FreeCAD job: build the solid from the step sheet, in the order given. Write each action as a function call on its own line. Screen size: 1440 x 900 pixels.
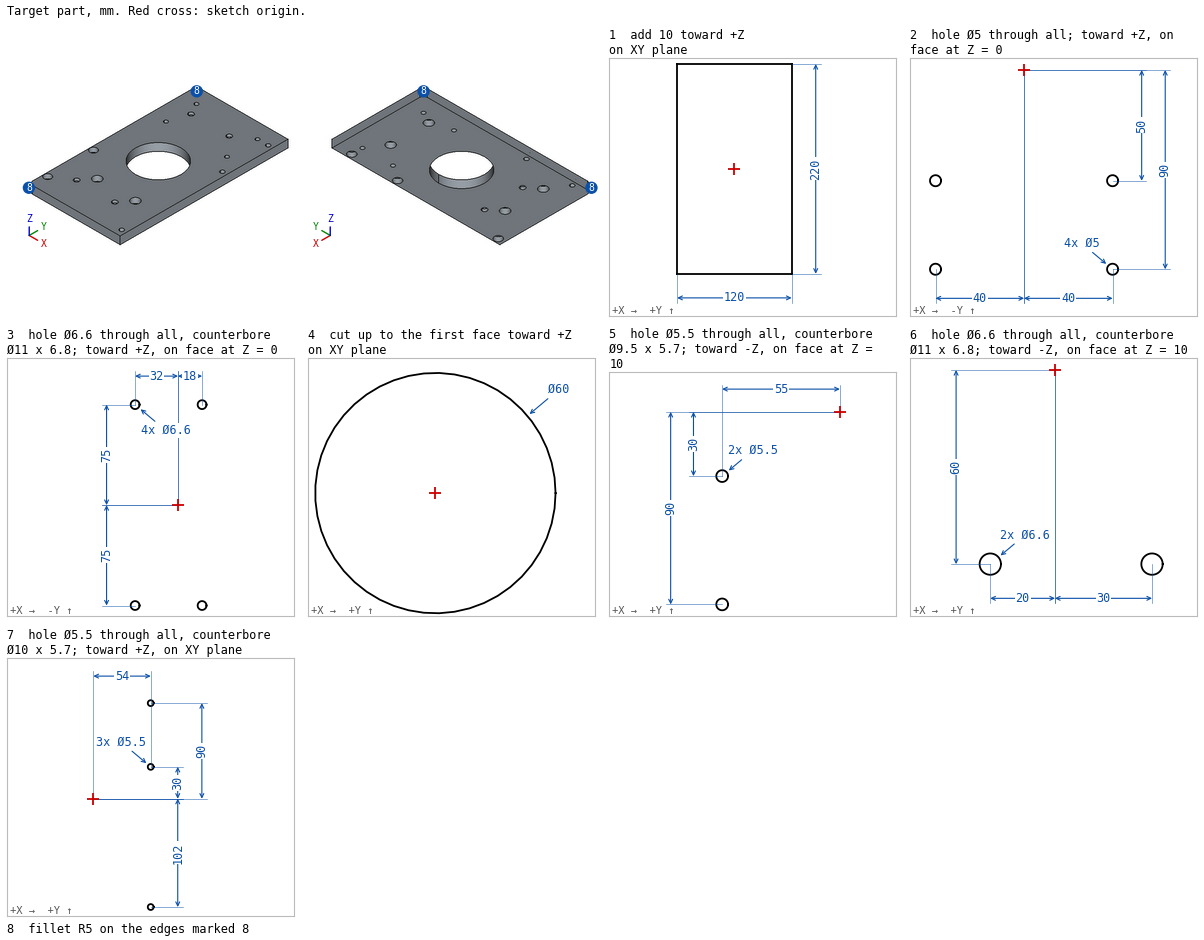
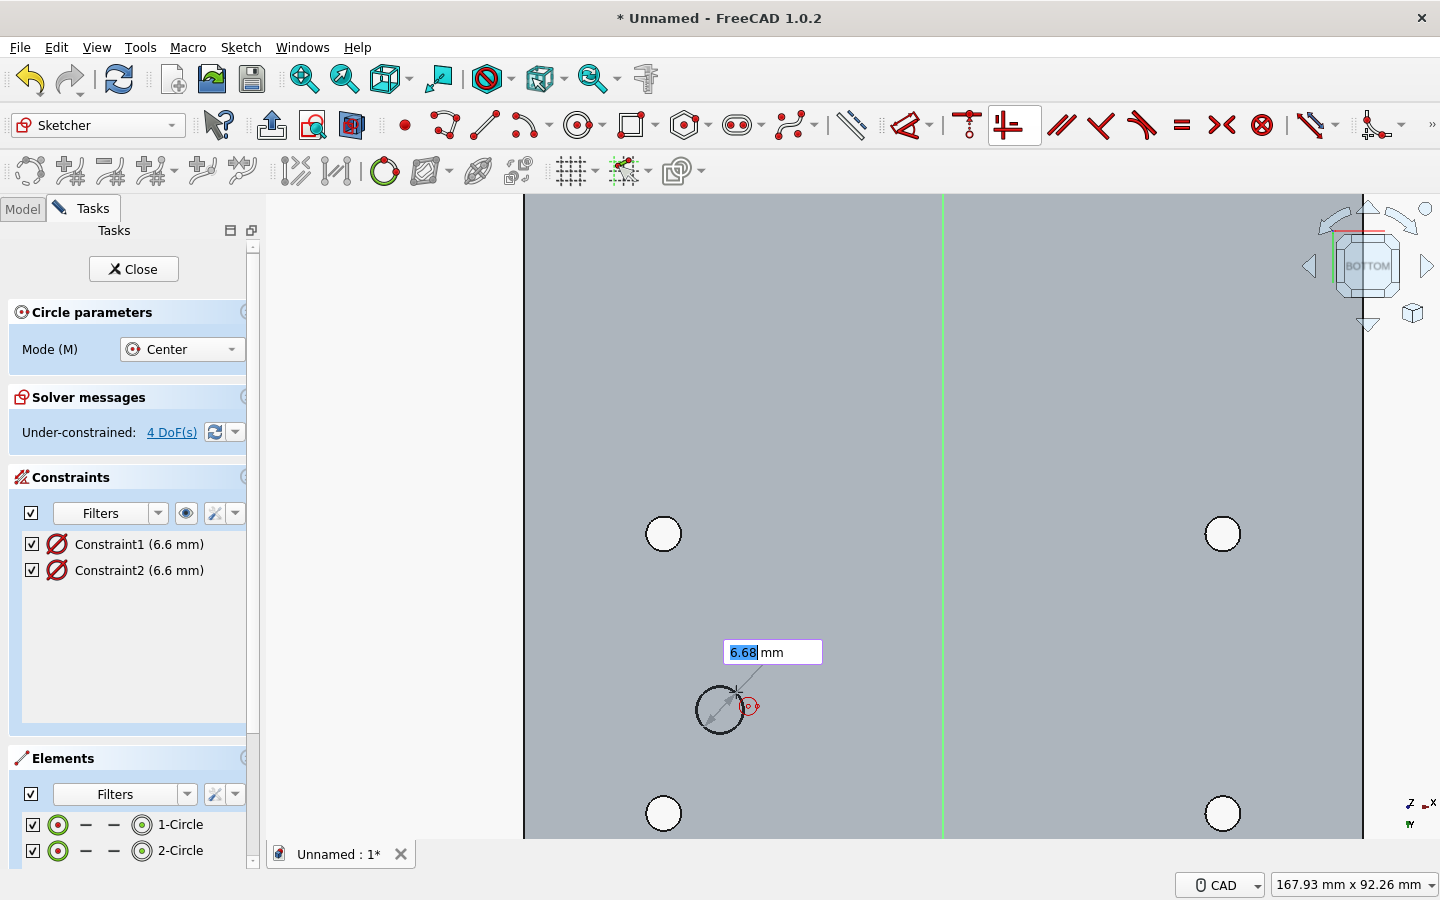
text(6.6)
key(Return)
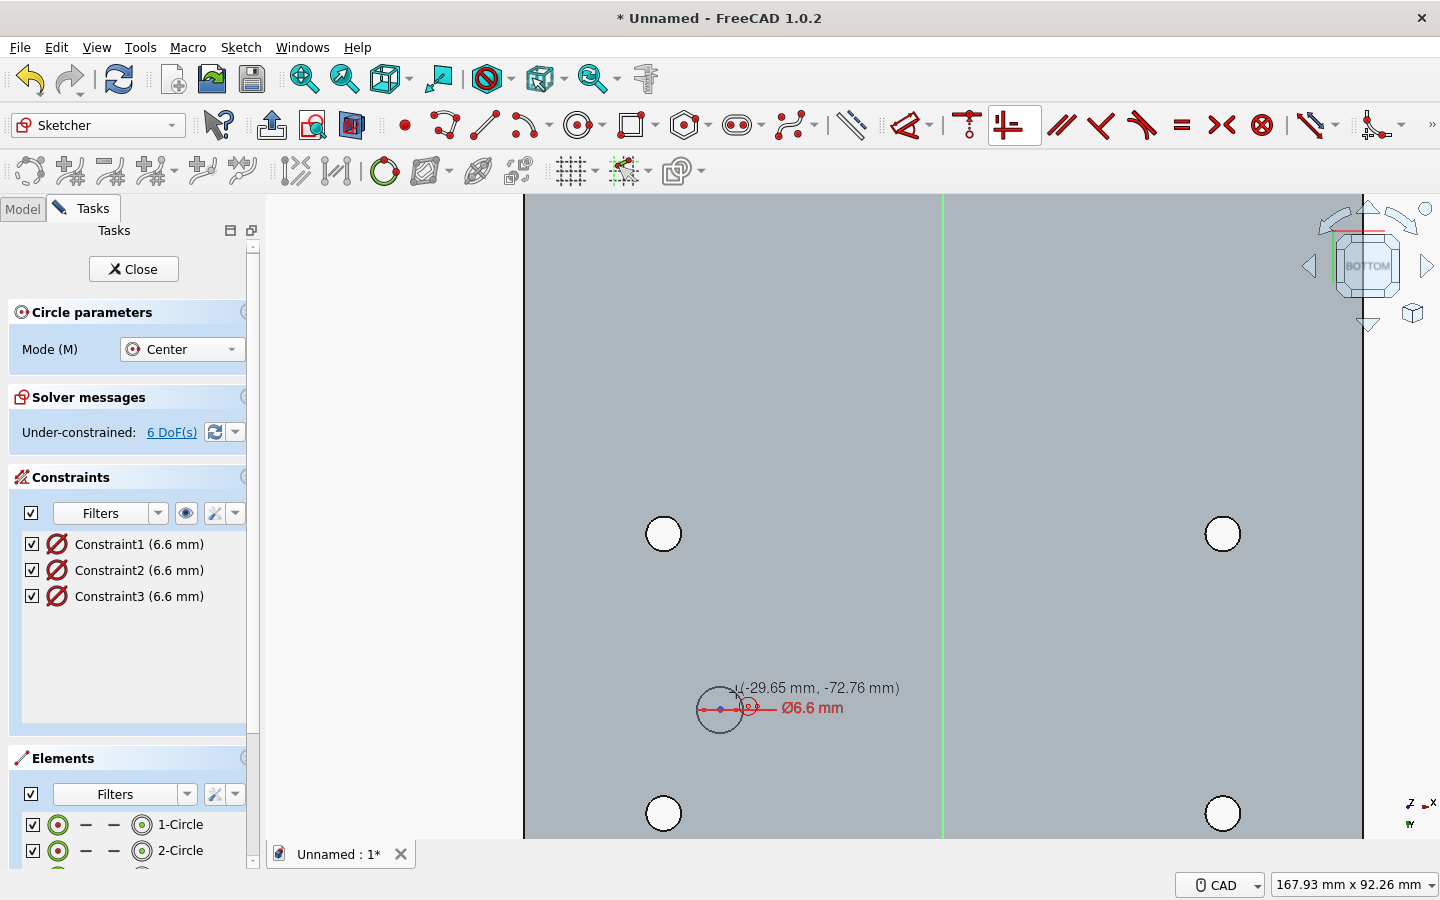
click(1069, 709)
move(1085, 692)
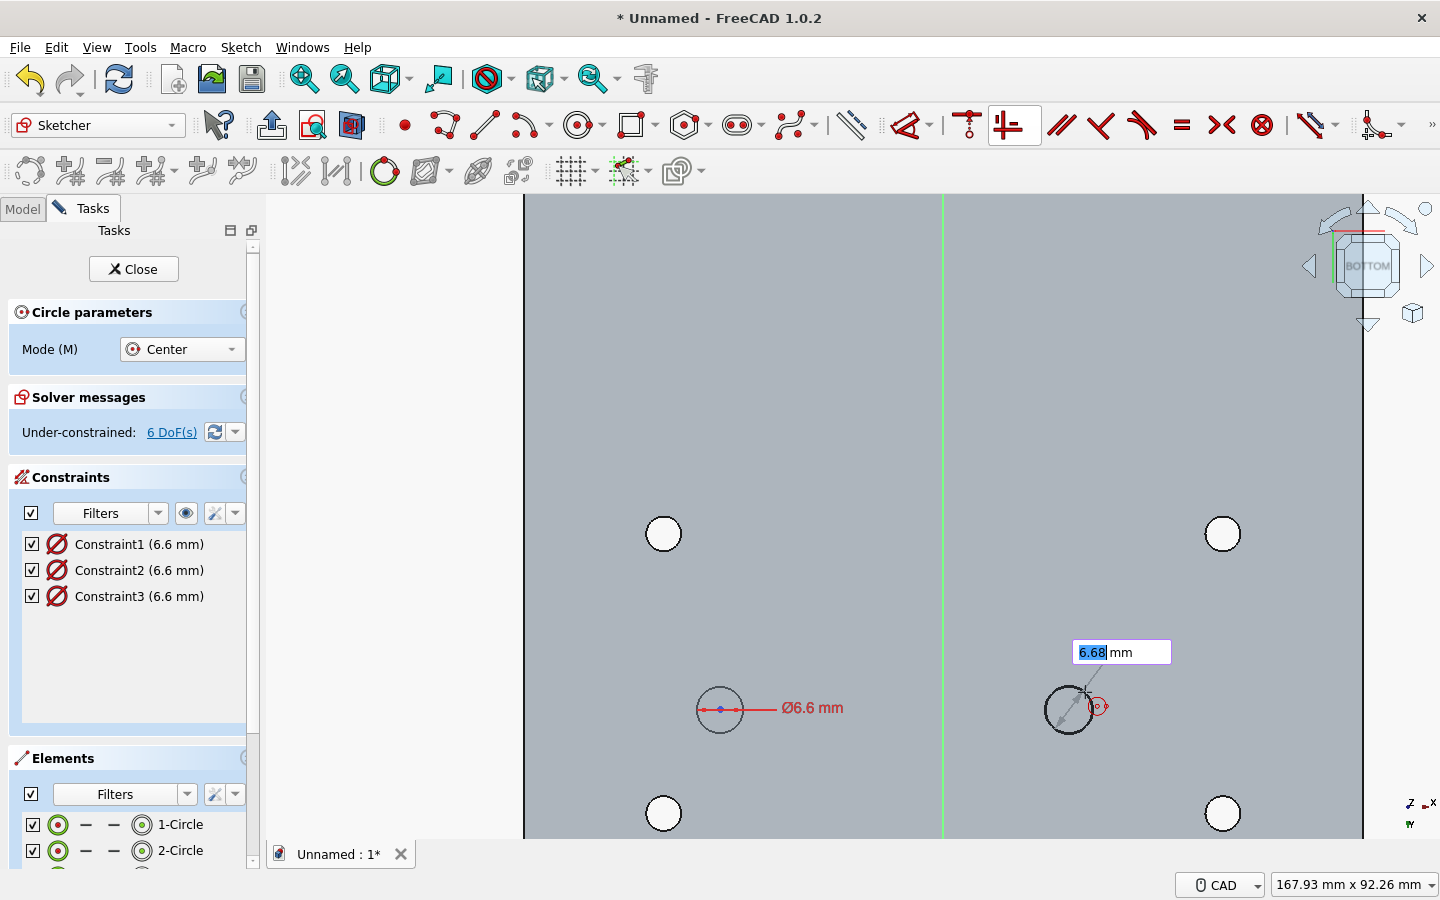
text(6.6)
key(Return)
key(Escape)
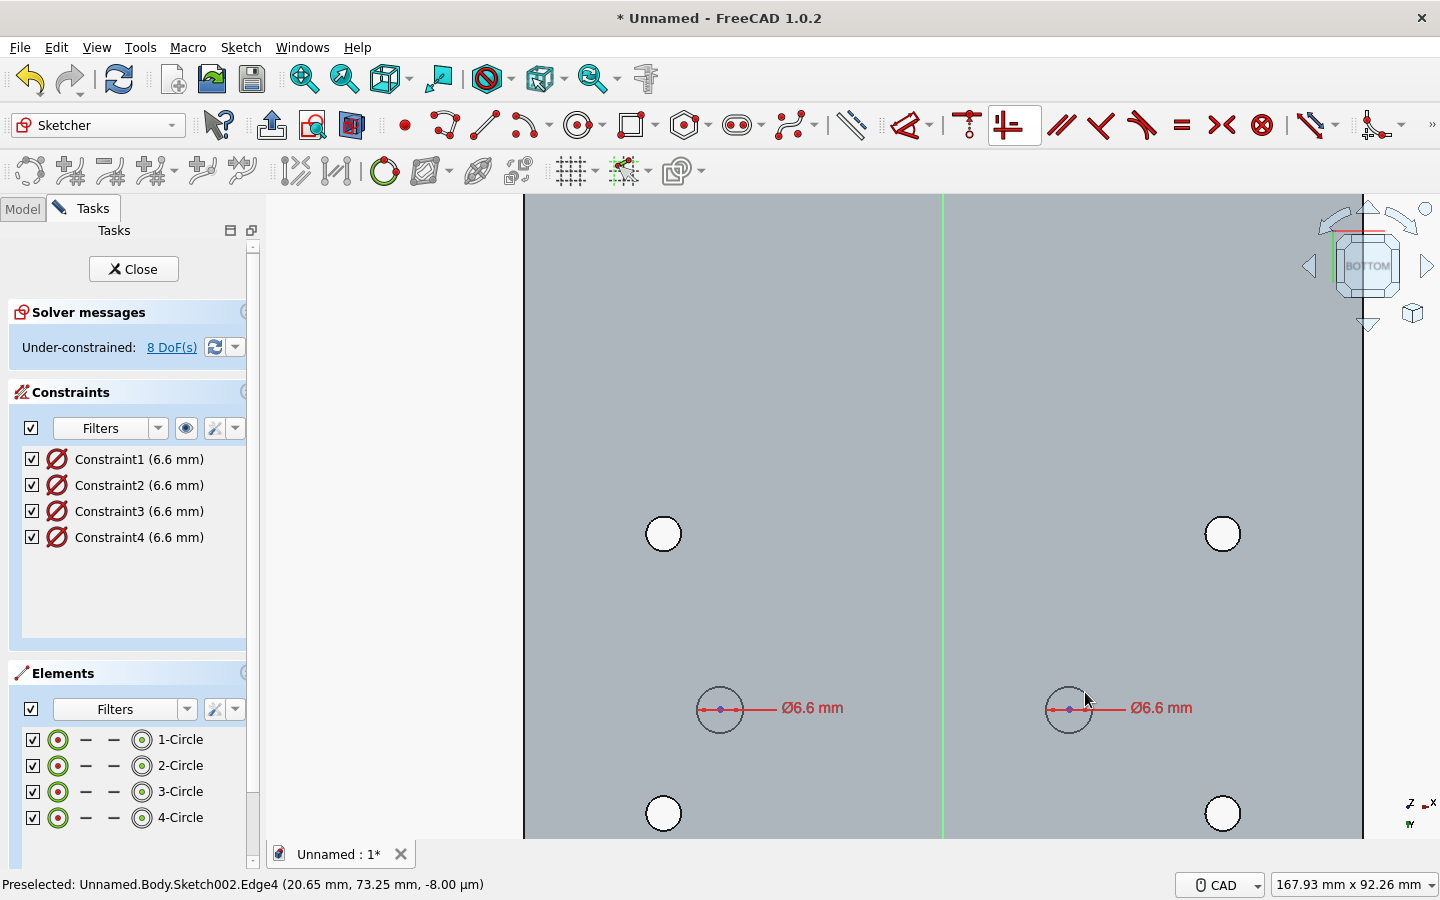
scroll(721, 710, down, 5)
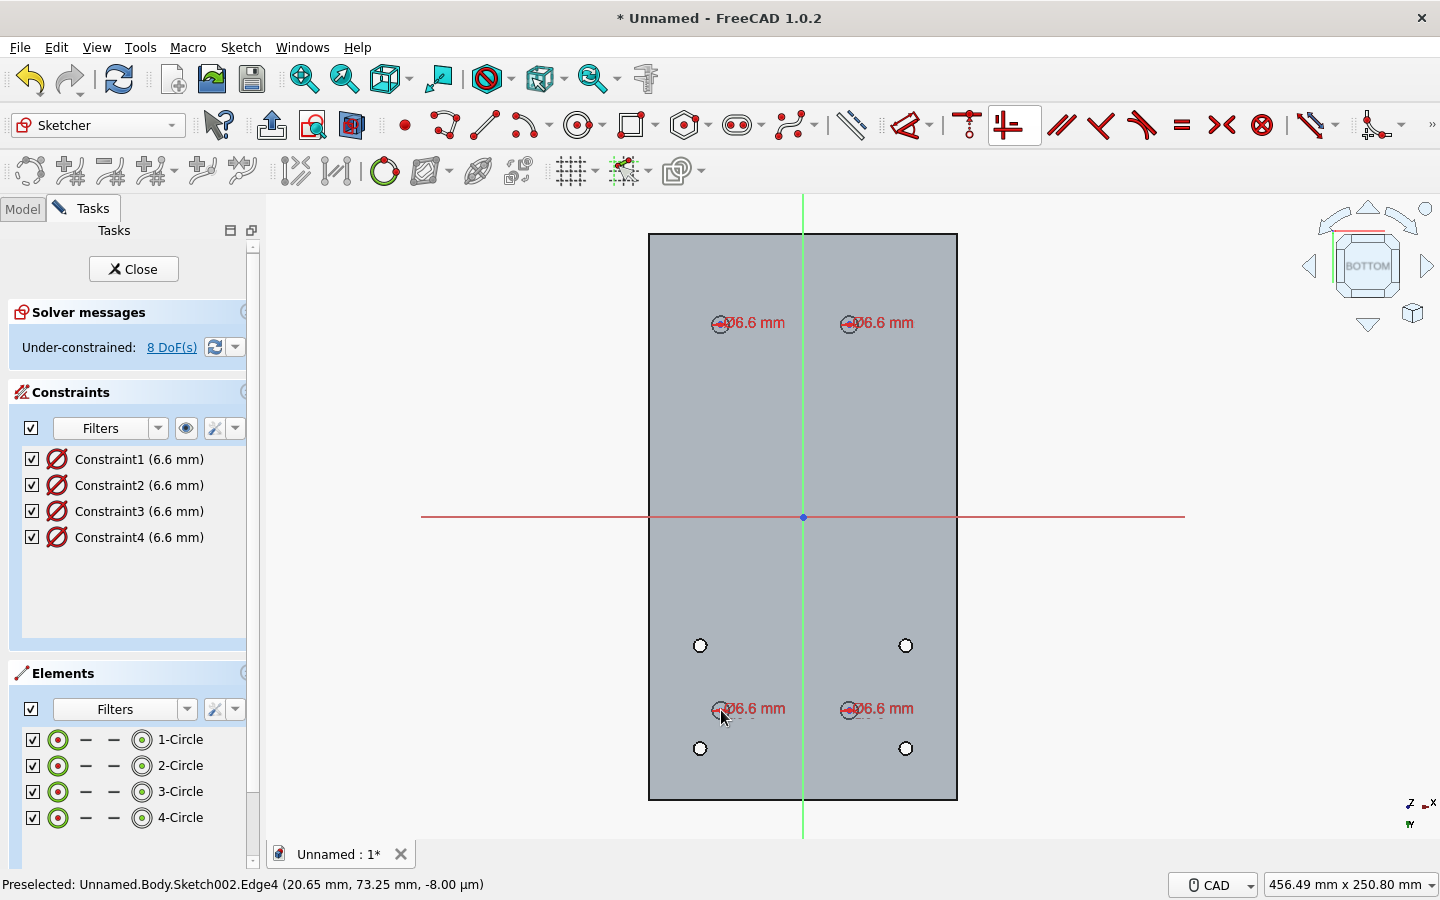
click(721, 325)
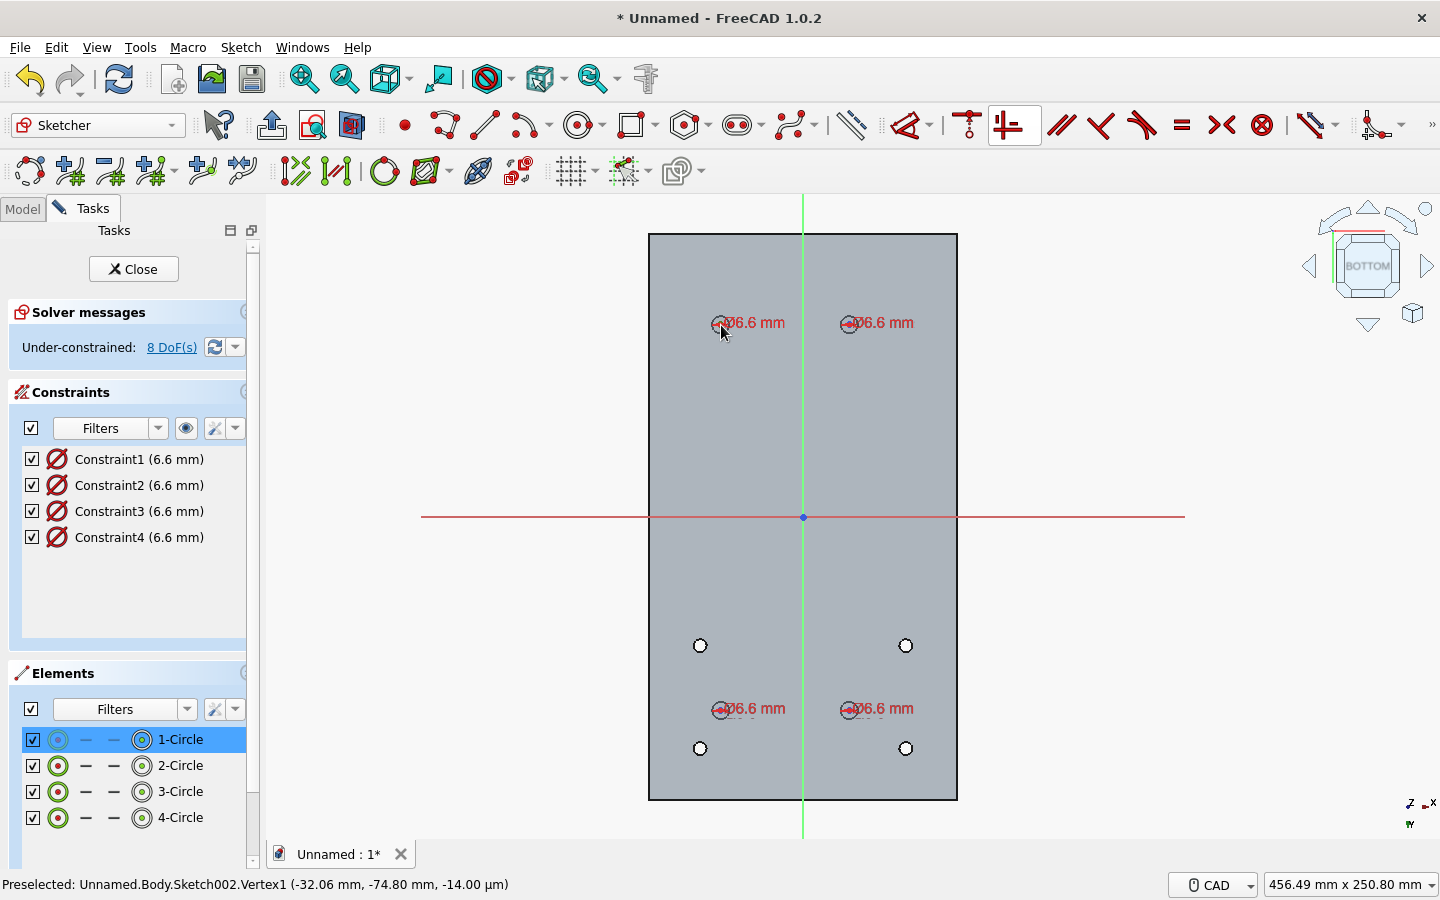
click(849, 325)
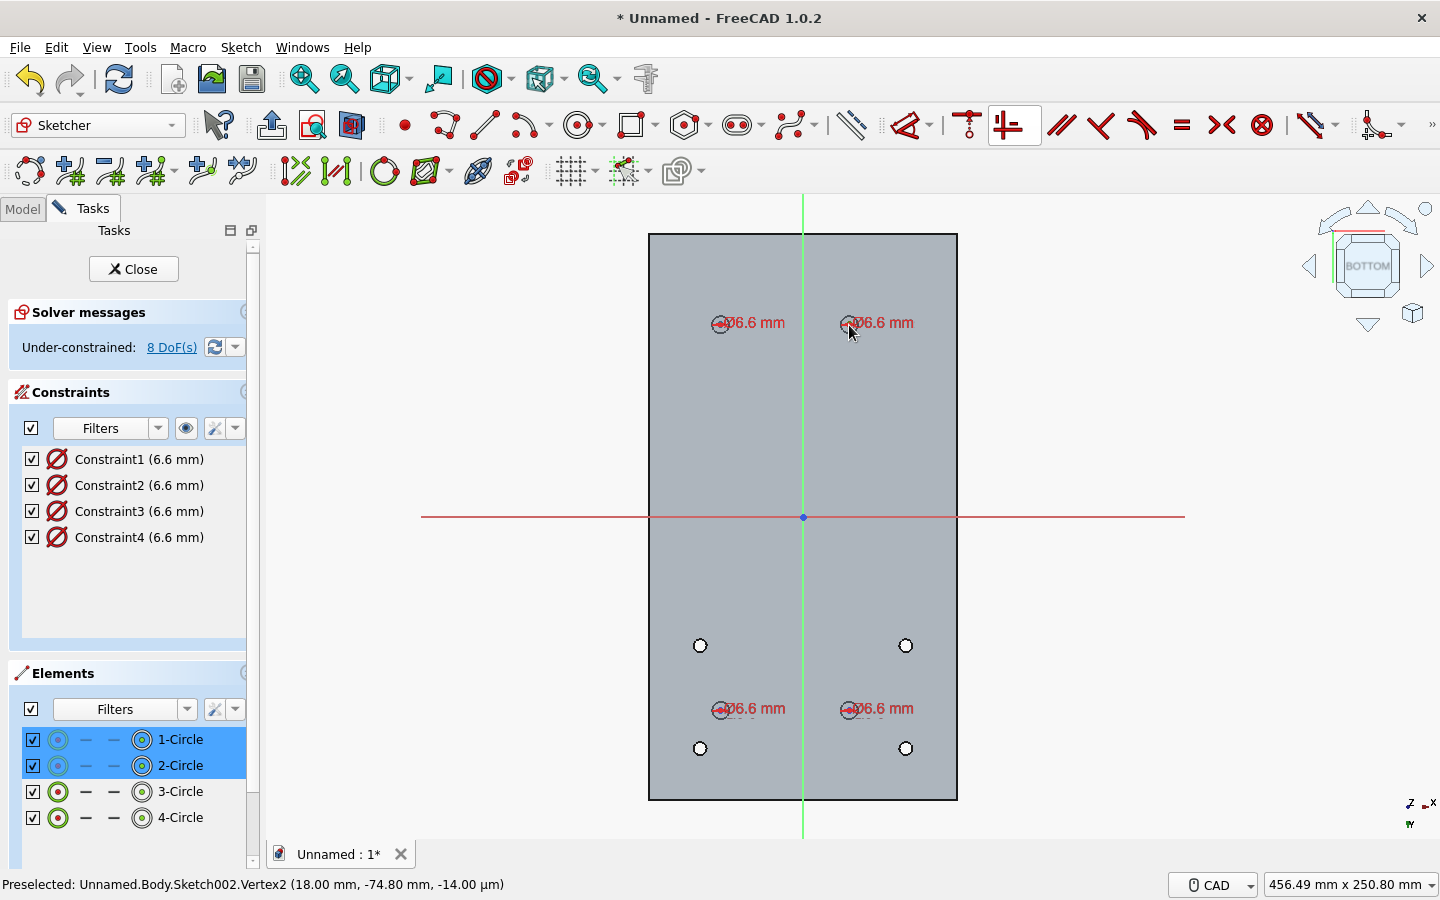
click(1036, 126)